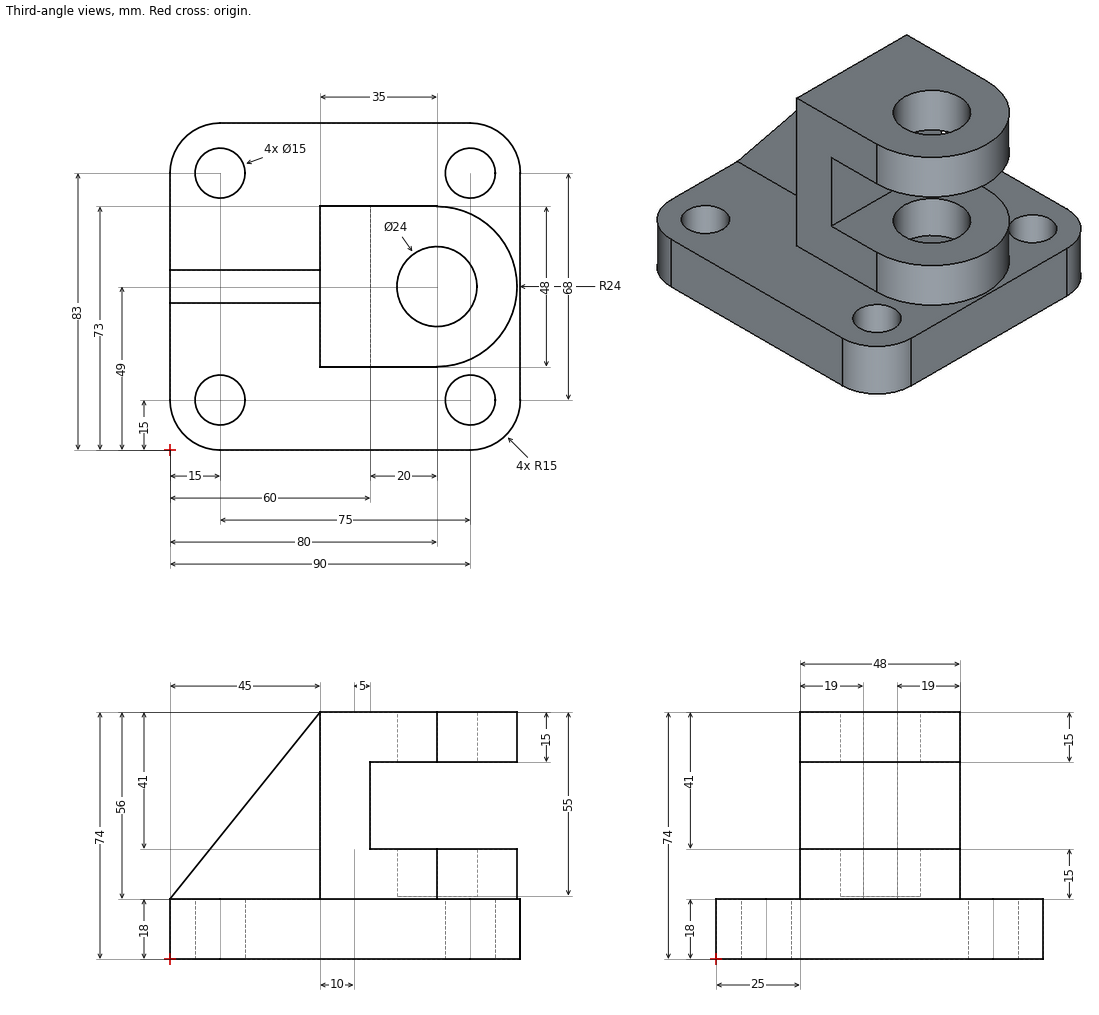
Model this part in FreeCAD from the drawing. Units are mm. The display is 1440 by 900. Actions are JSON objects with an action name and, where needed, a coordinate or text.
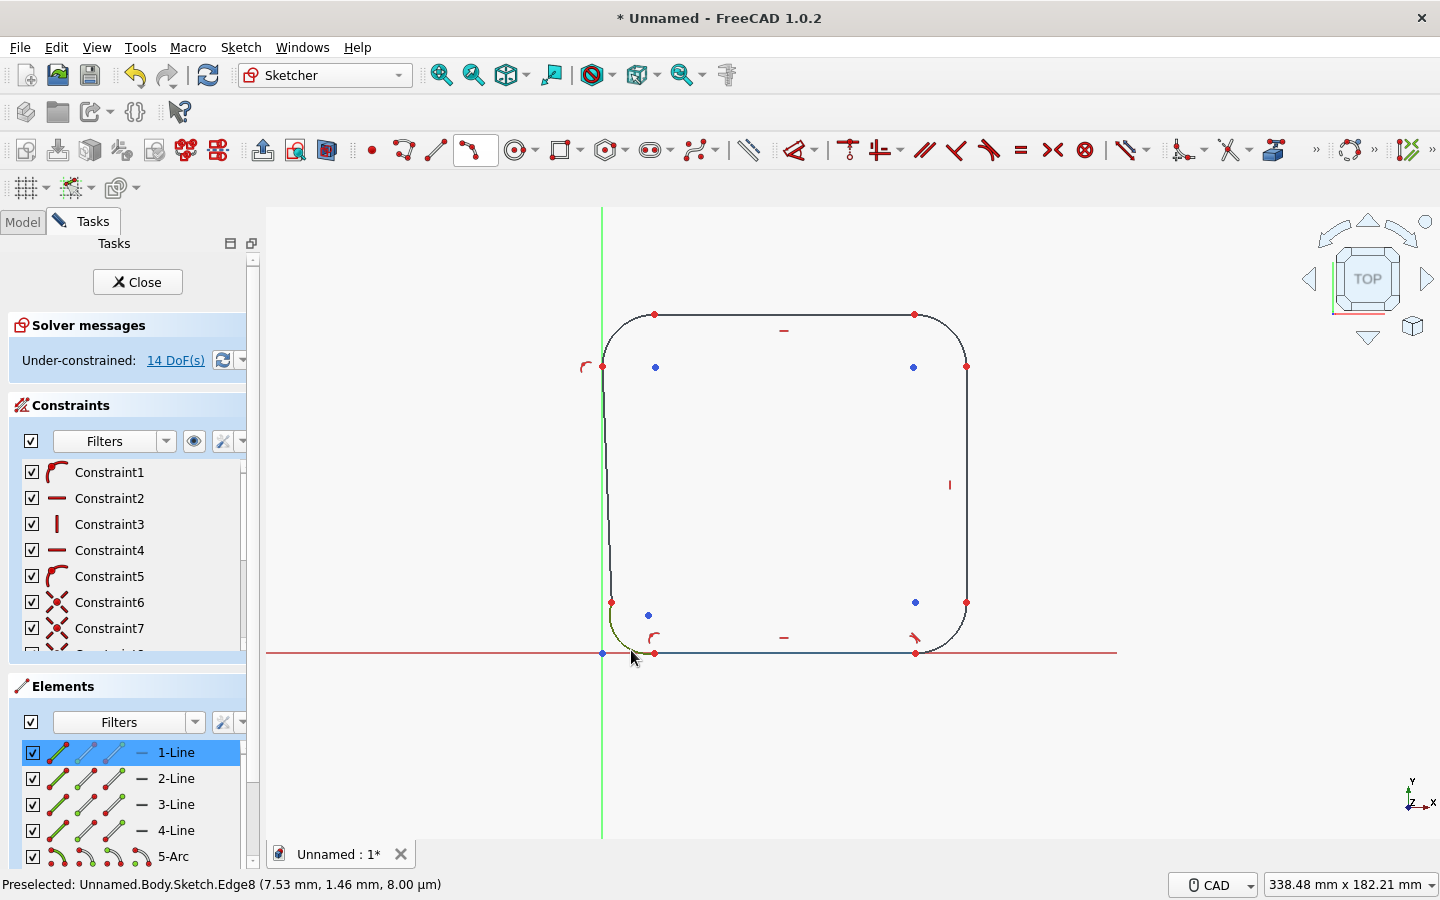
{"action": "left_click", "coordinate": [990, 150]}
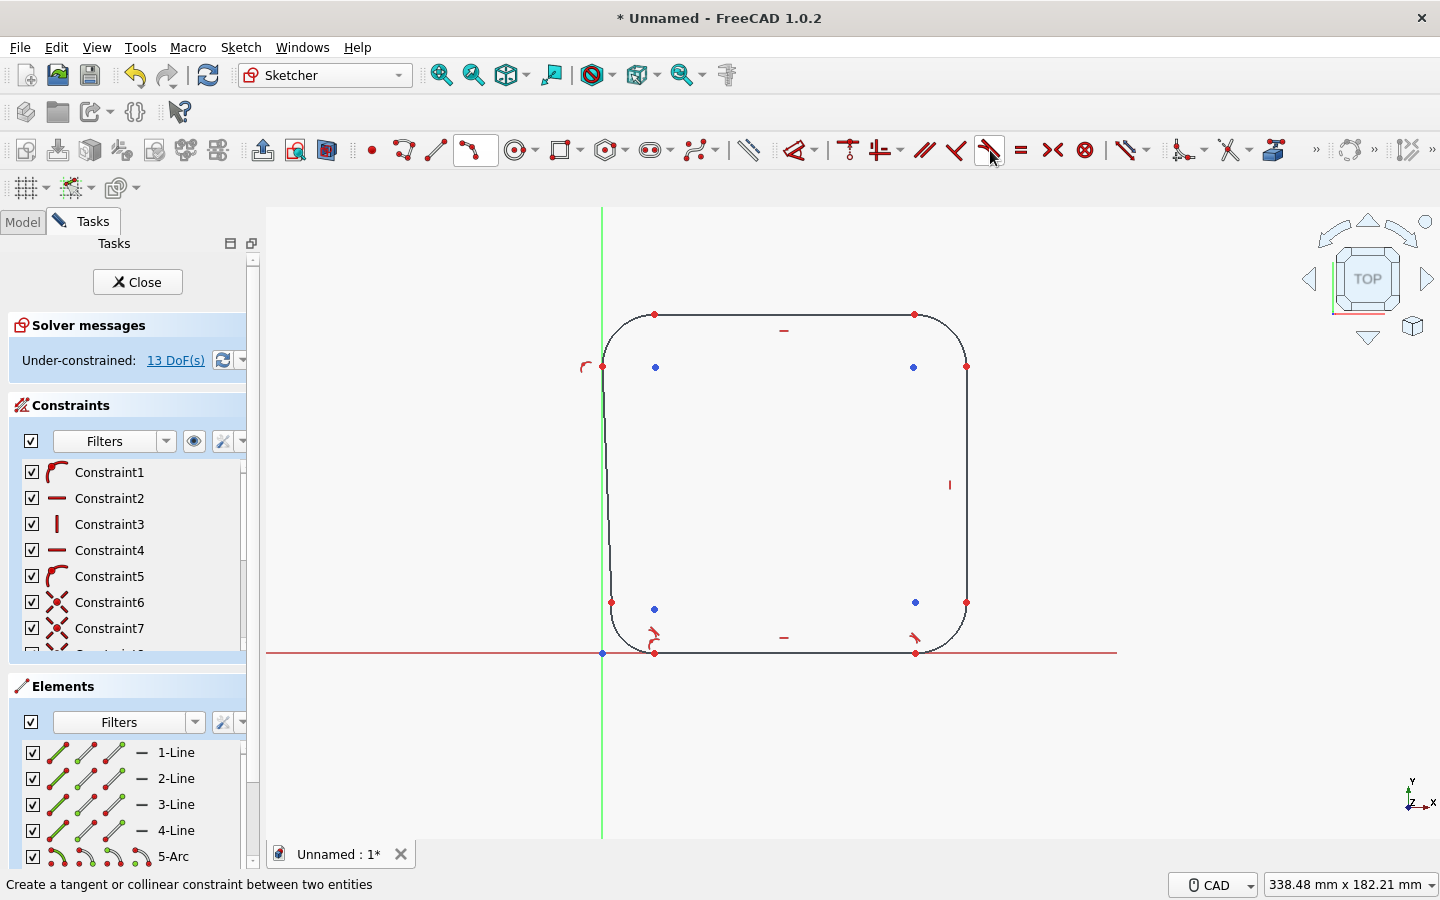
{"action": "left_click", "coordinate": [967, 532]}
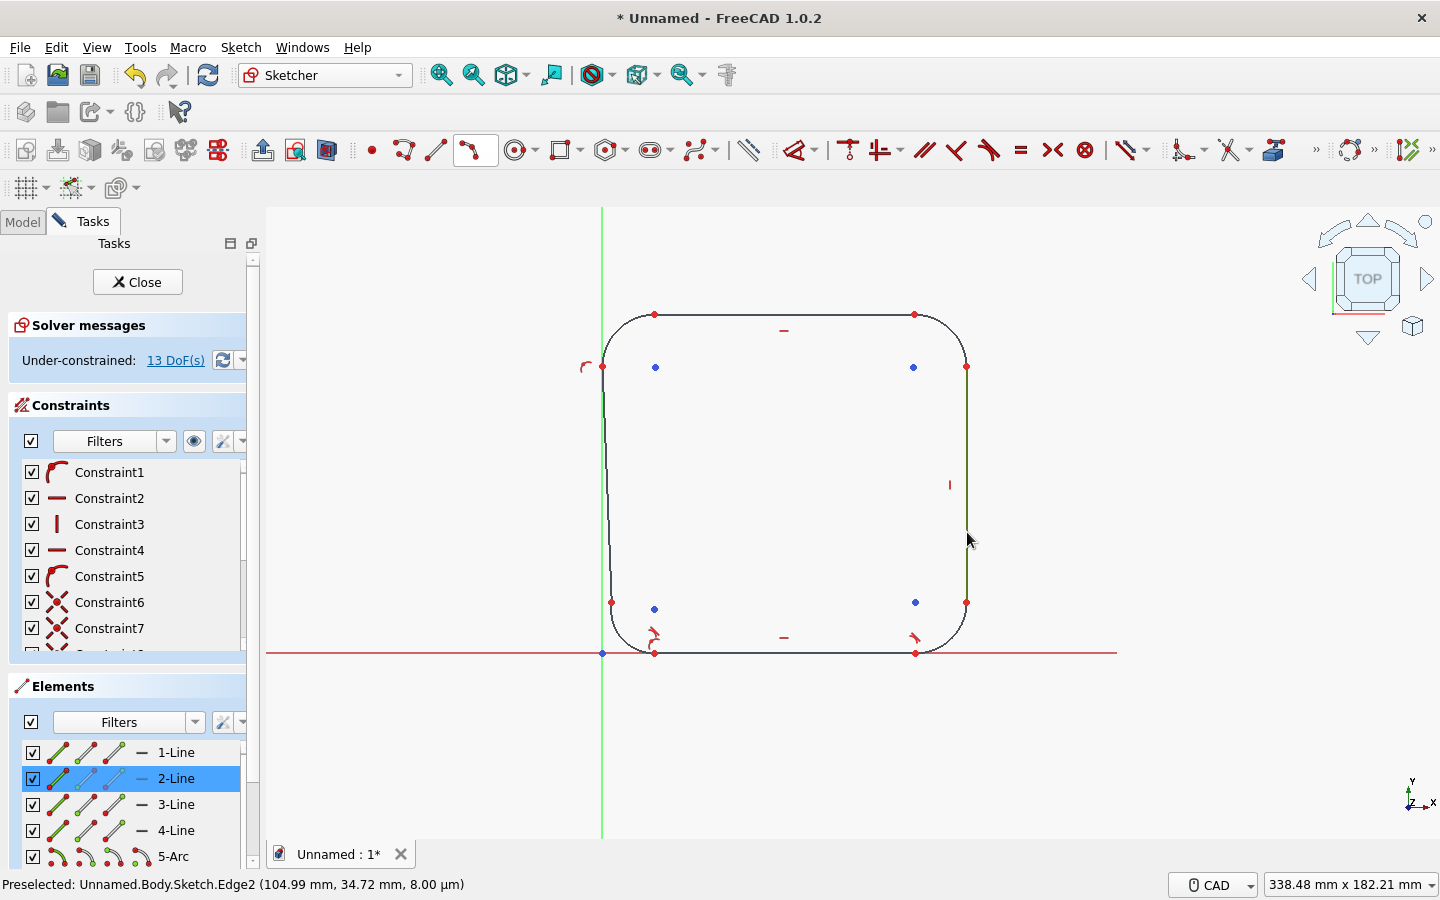
{"action": "left_click", "coordinate": [961, 626]}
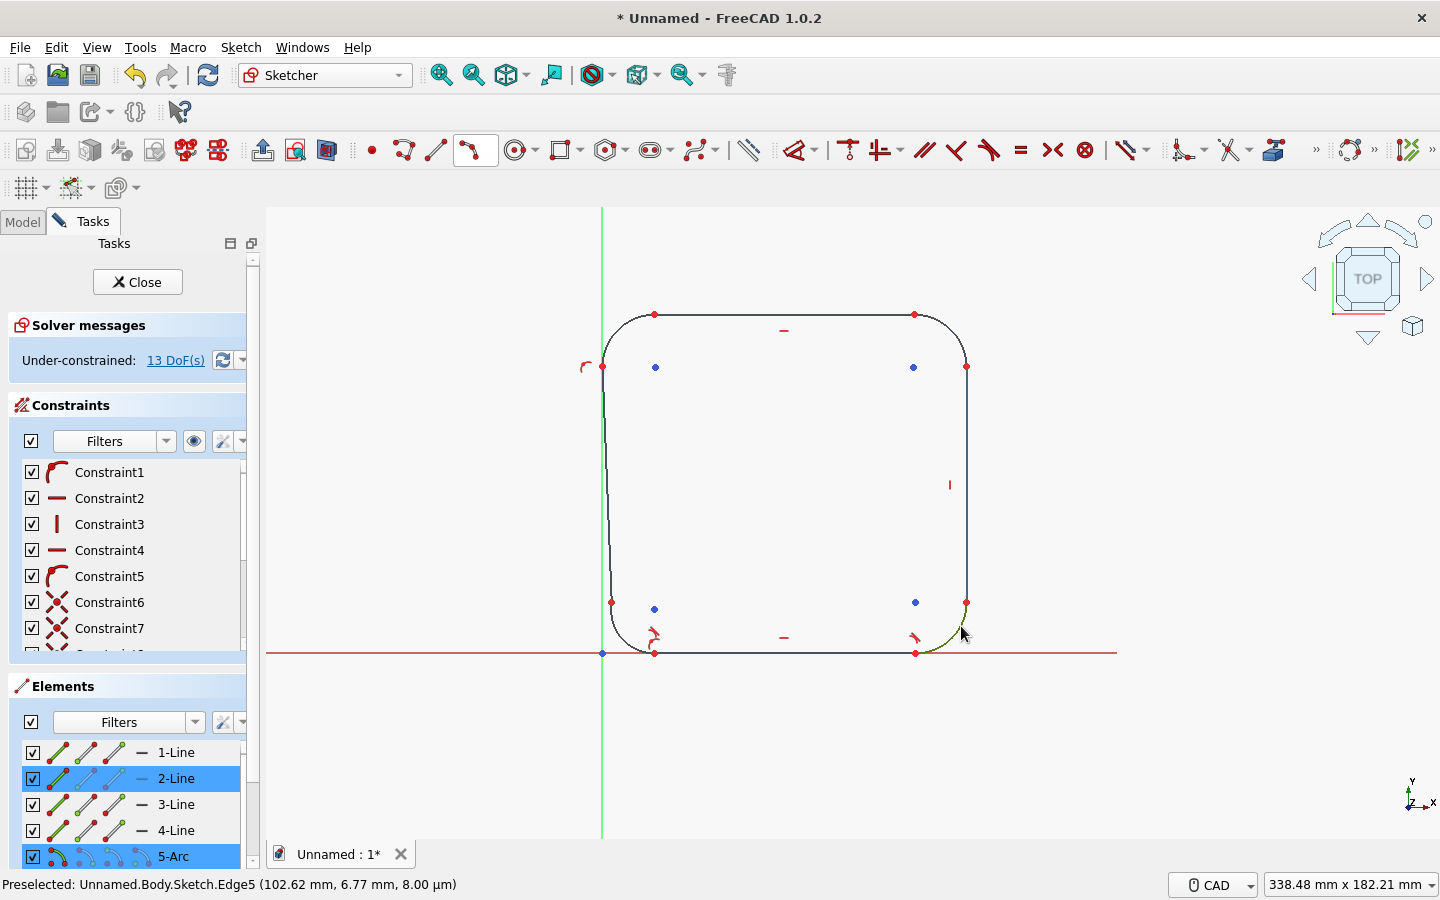
{"action": "left_click", "coordinate": [990, 150]}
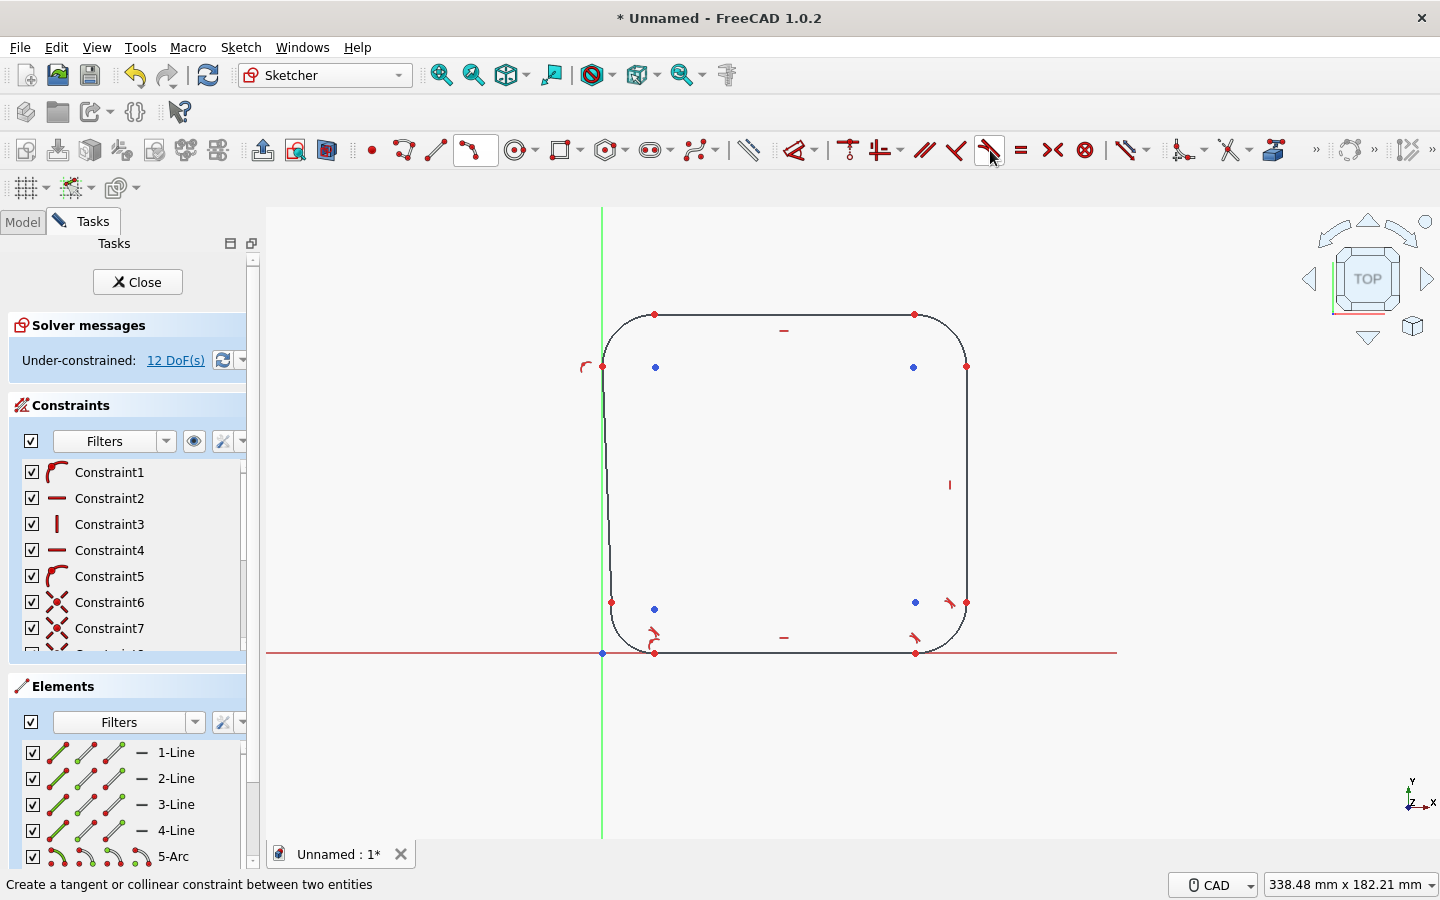
{"action": "left_click", "coordinate": [967, 531]}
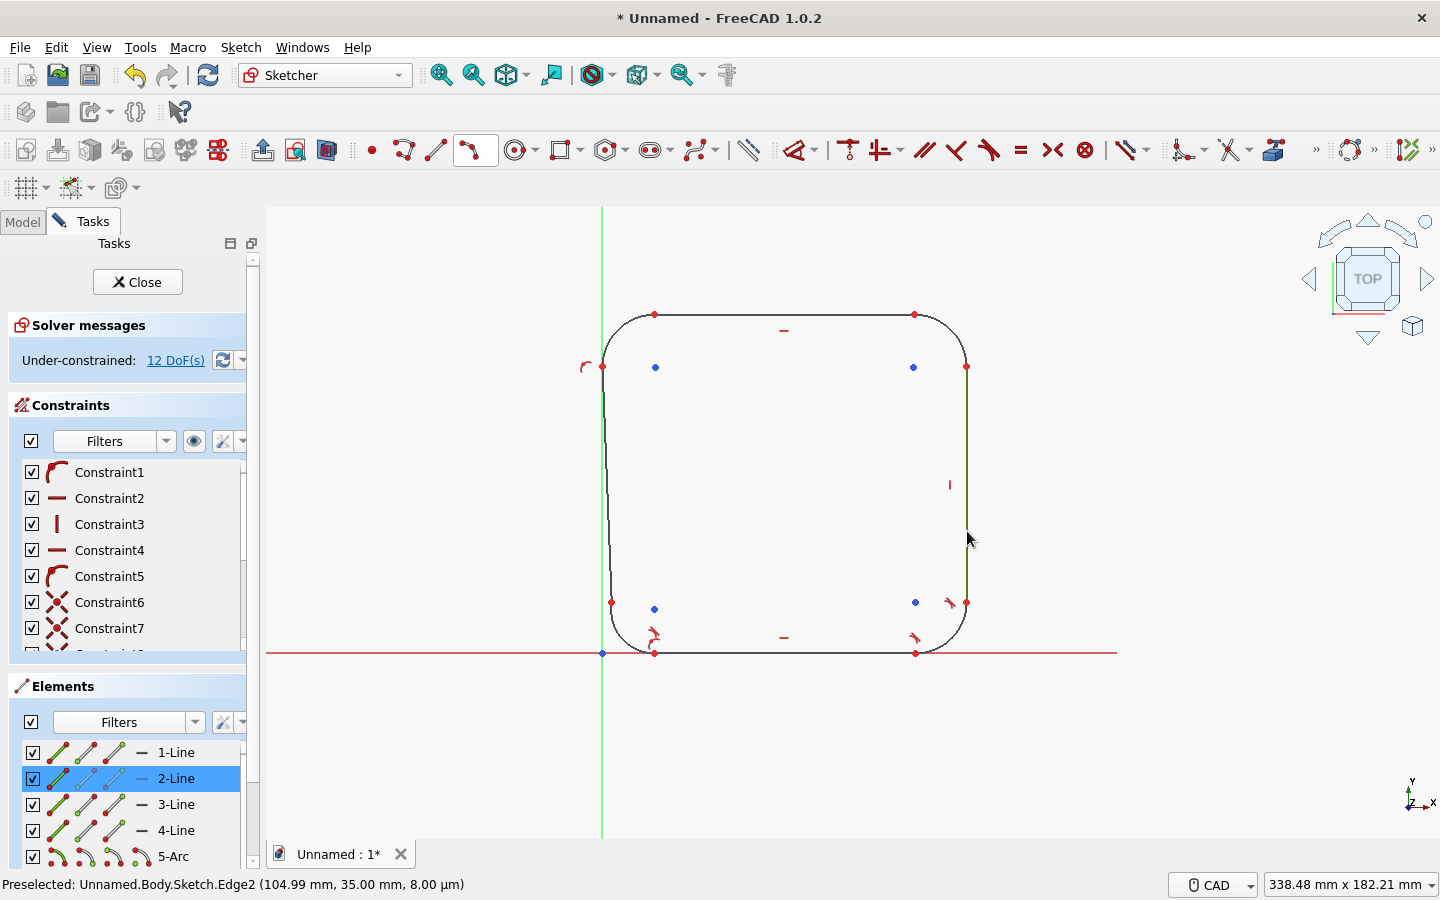
{"action": "left_click", "coordinate": [961, 343]}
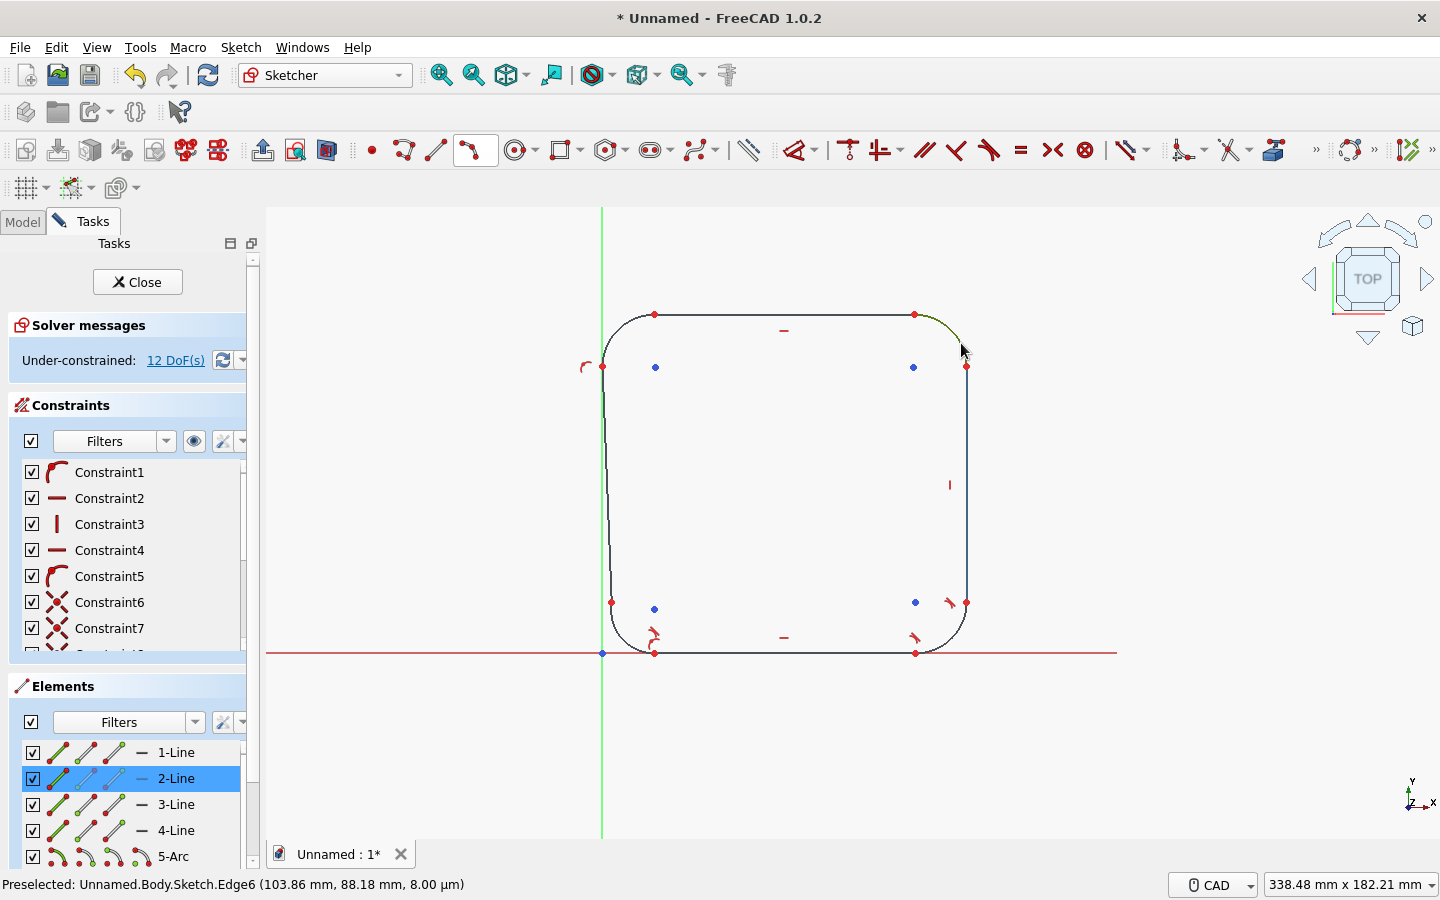
{"action": "left_click", "coordinate": [990, 150]}